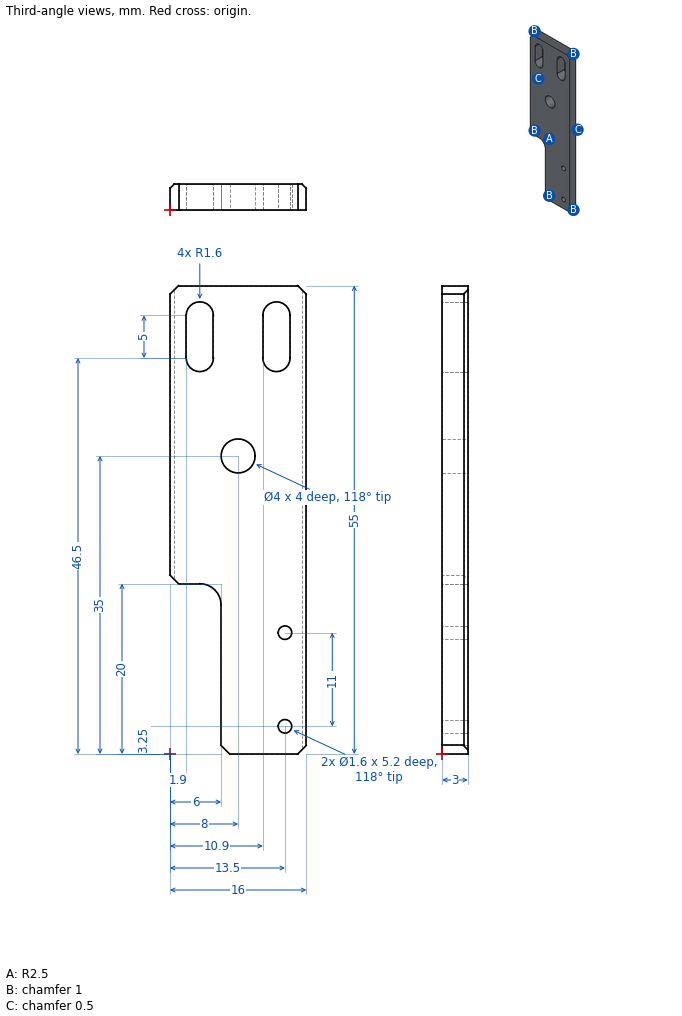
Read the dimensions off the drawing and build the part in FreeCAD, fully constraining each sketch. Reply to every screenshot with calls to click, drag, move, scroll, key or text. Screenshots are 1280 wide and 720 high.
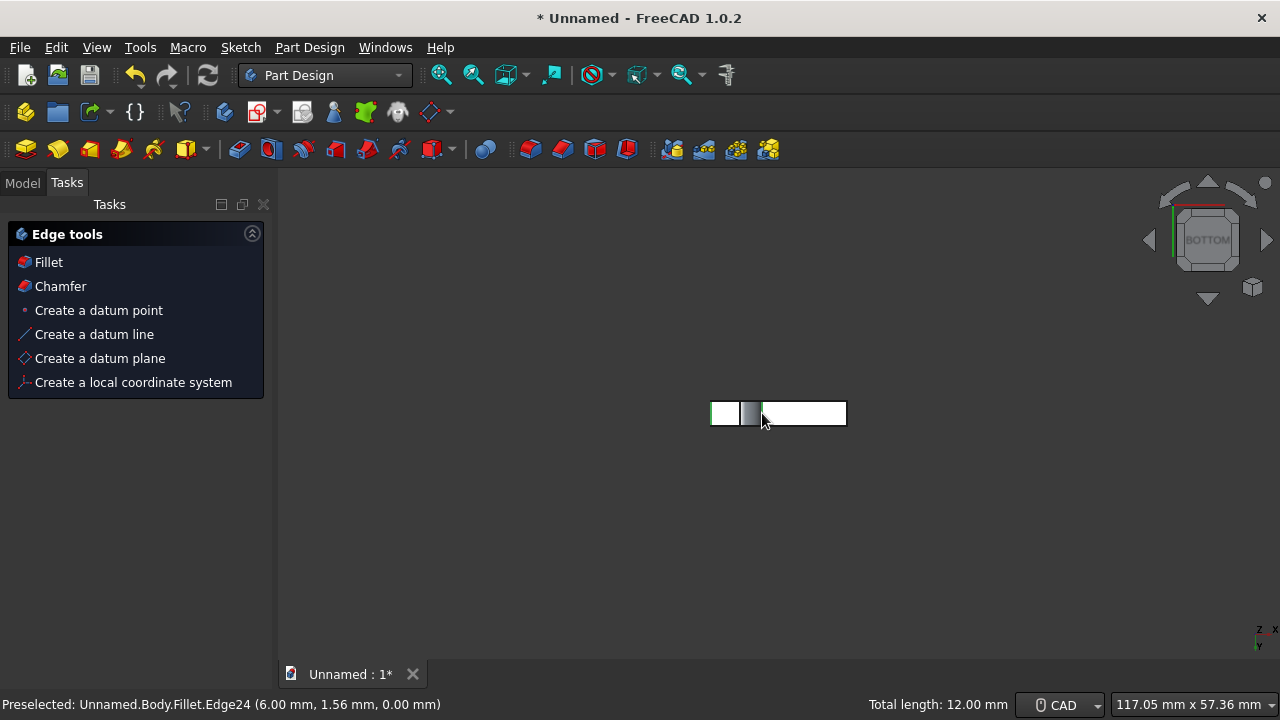
click(847, 413, ctrl)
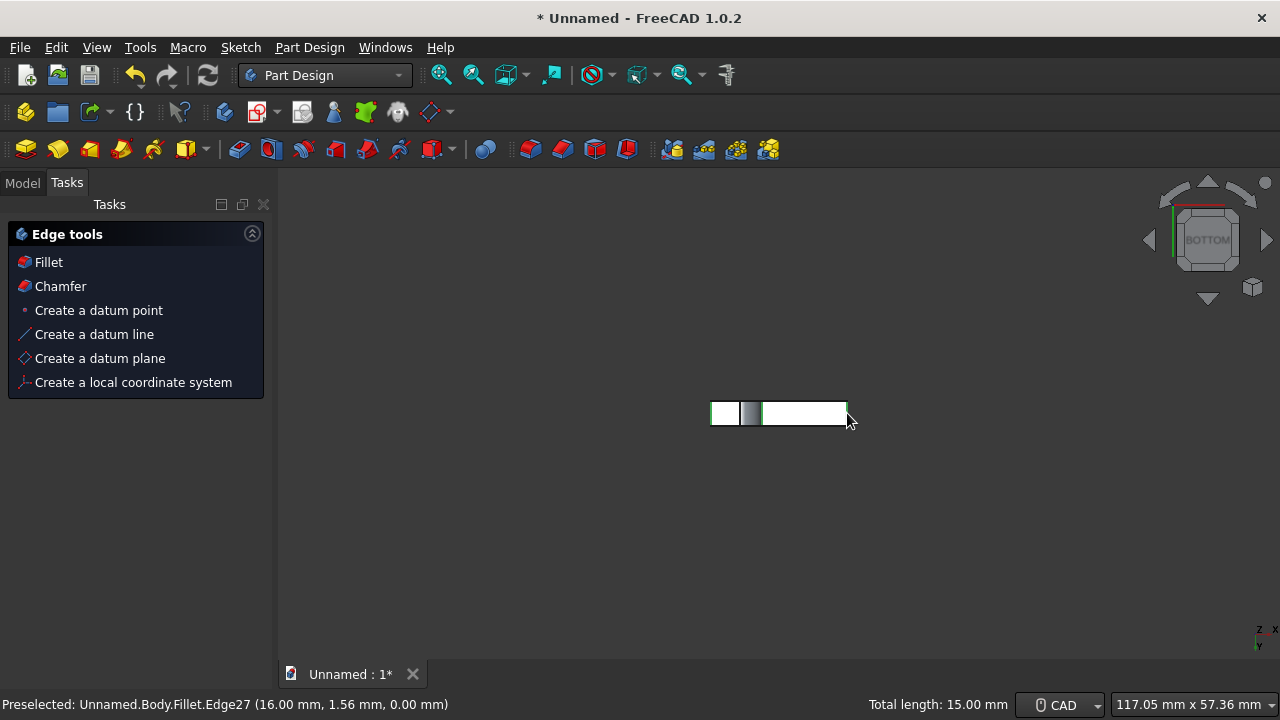
click(564, 150)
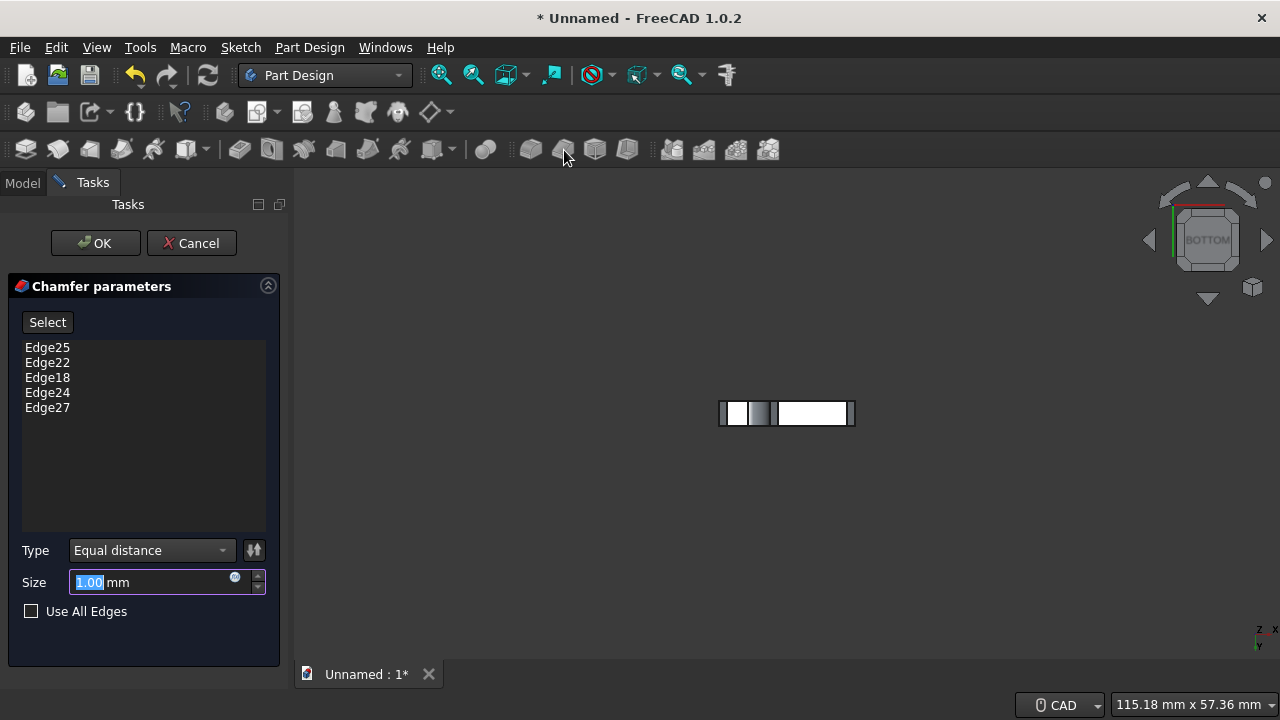
text(1)
key(Tab)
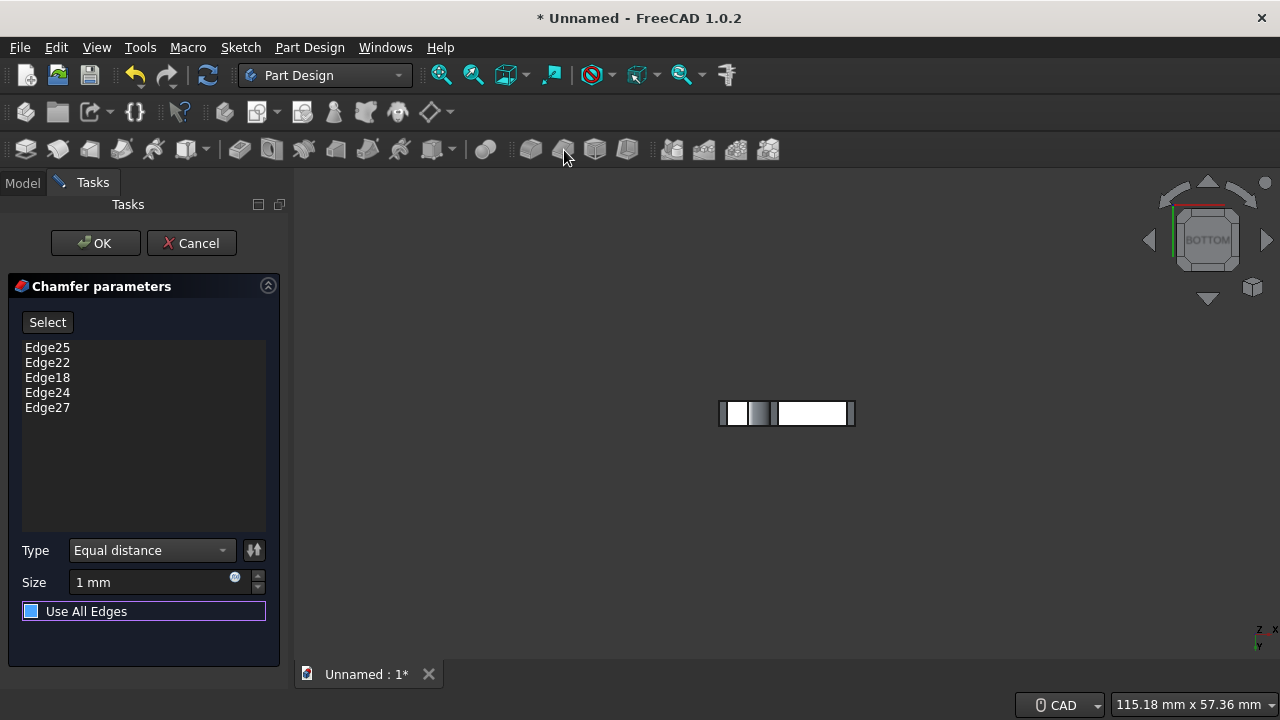
click(96, 243)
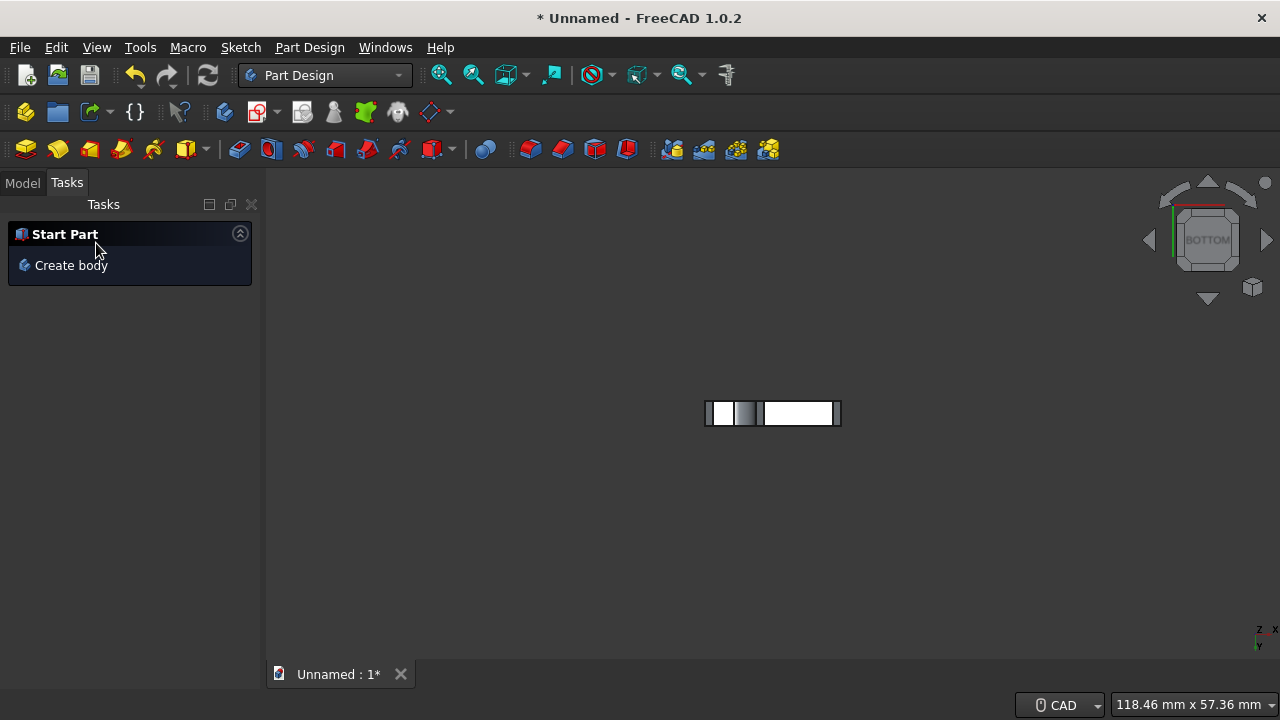
click(442, 76)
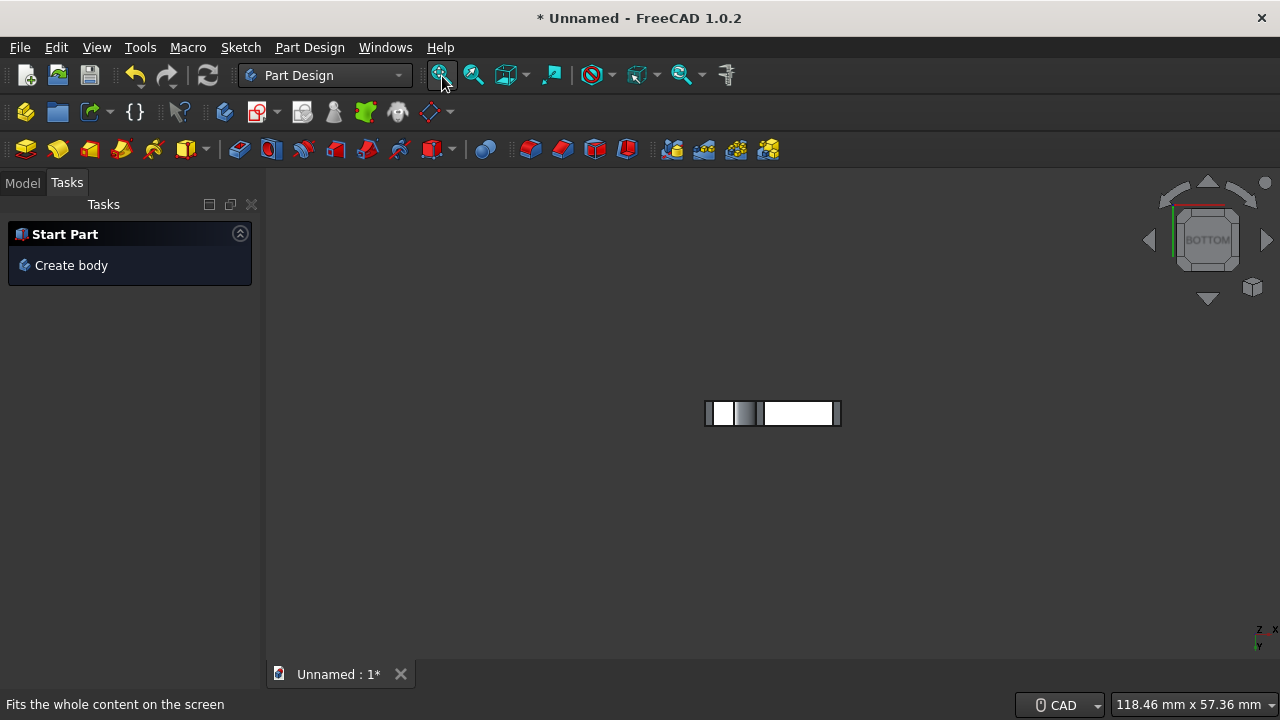
key(0)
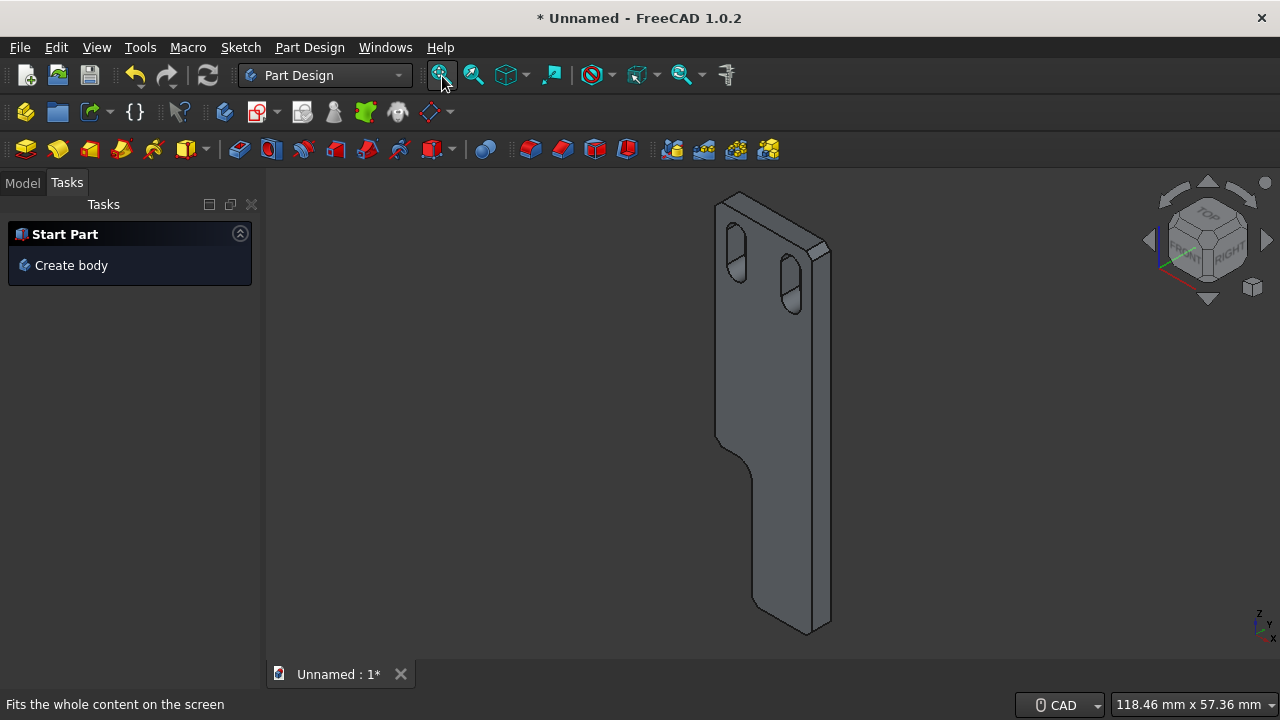
key(2)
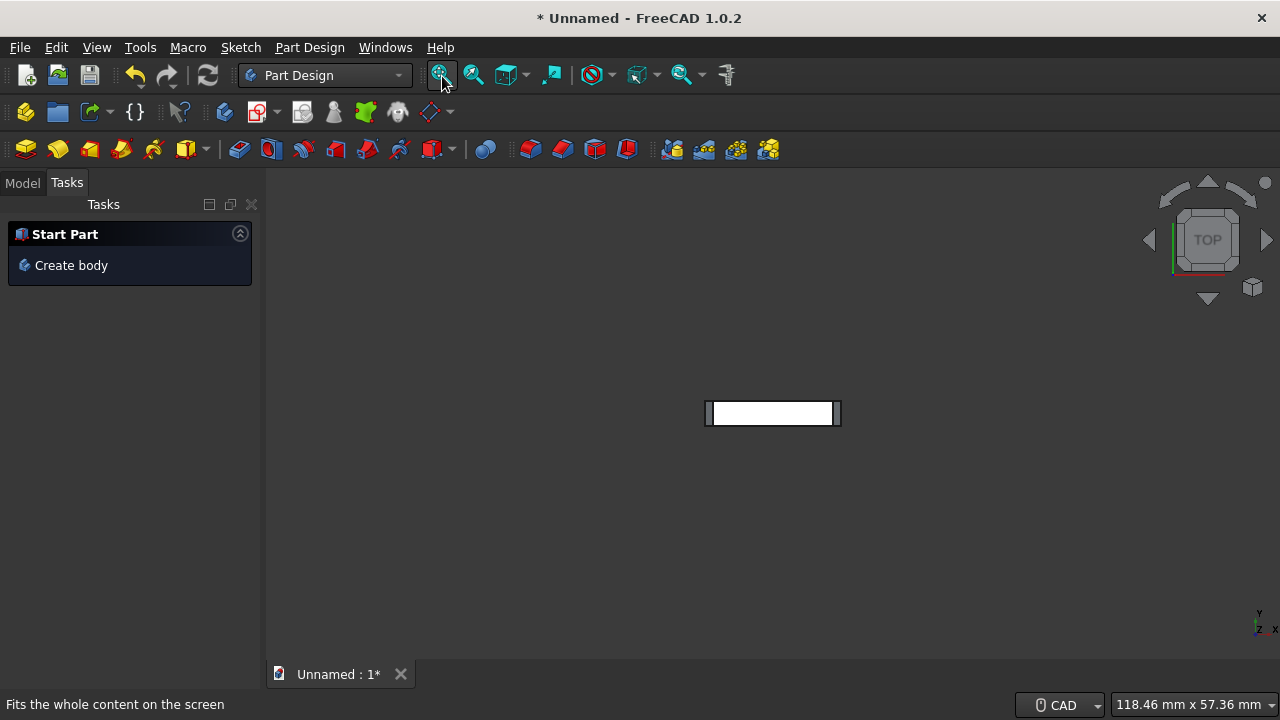
click(442, 76)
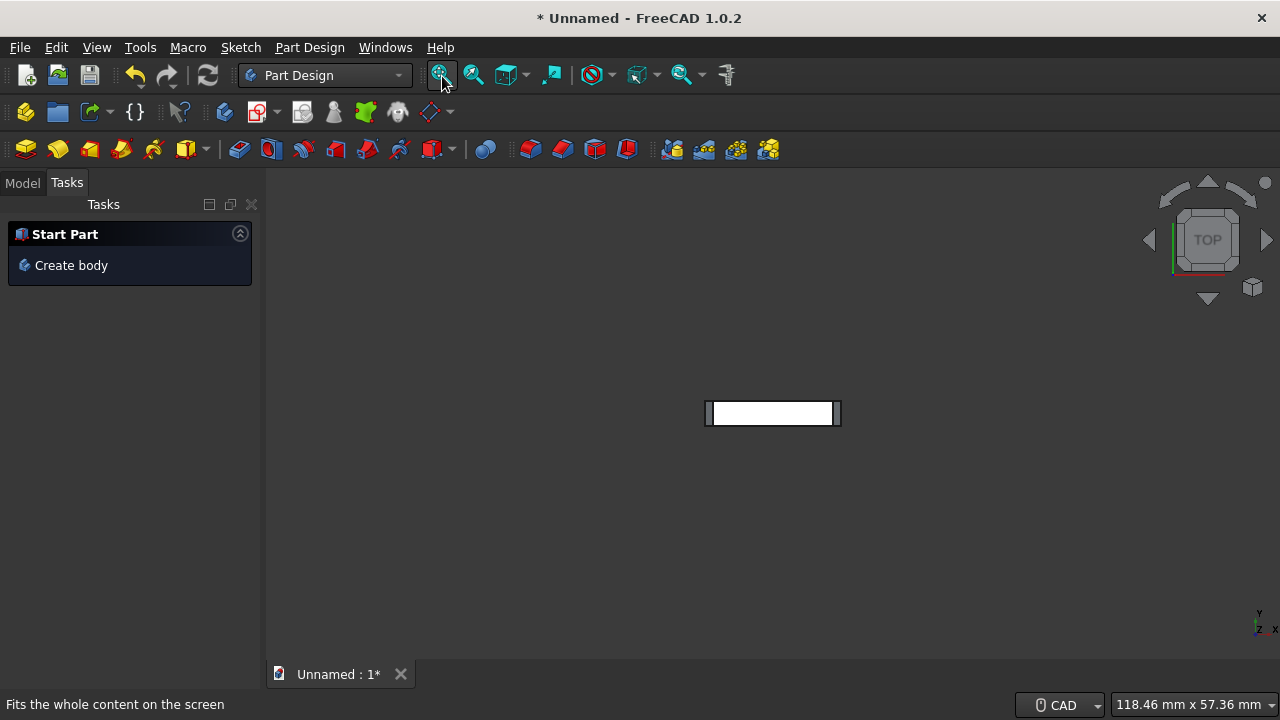
key(1)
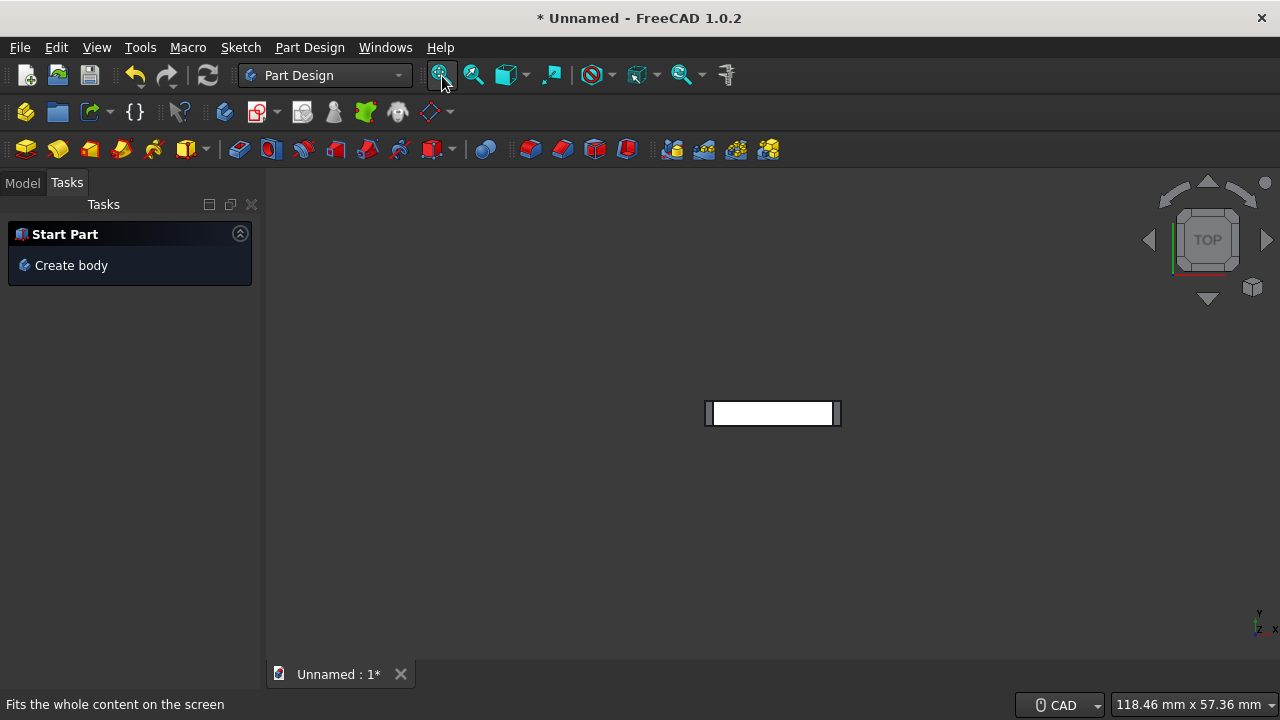
key(3)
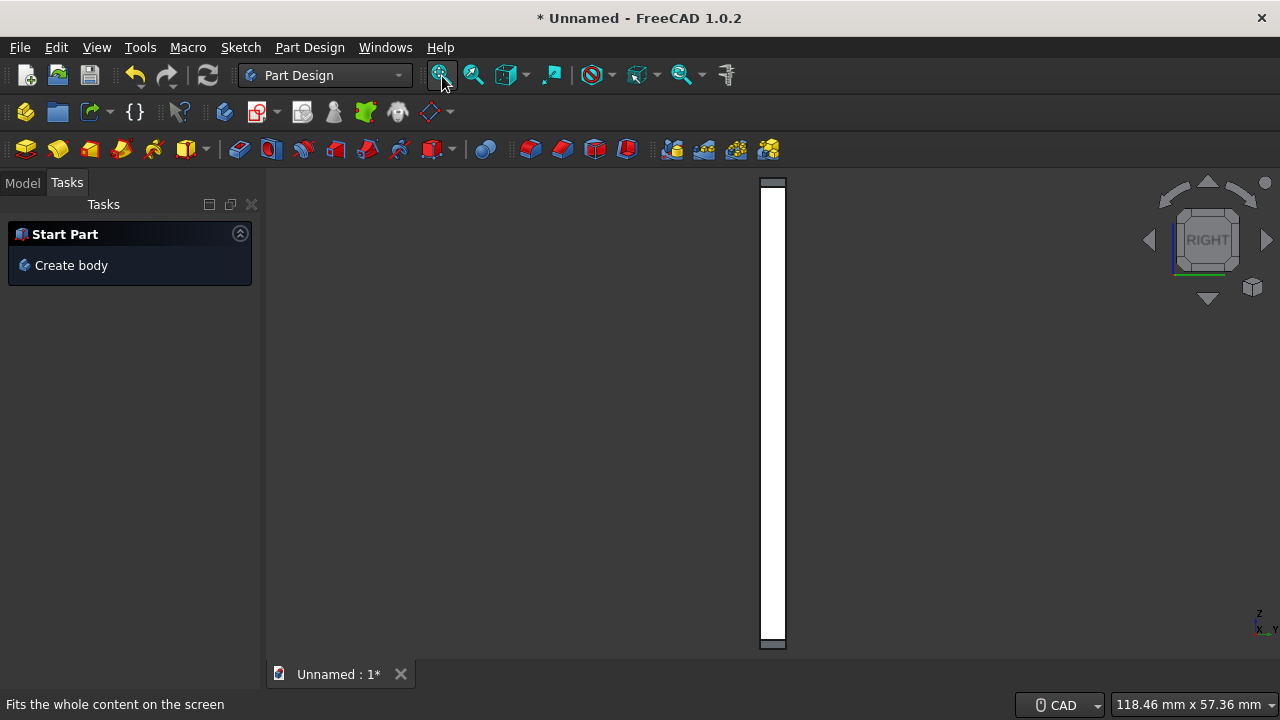
click(786, 413)